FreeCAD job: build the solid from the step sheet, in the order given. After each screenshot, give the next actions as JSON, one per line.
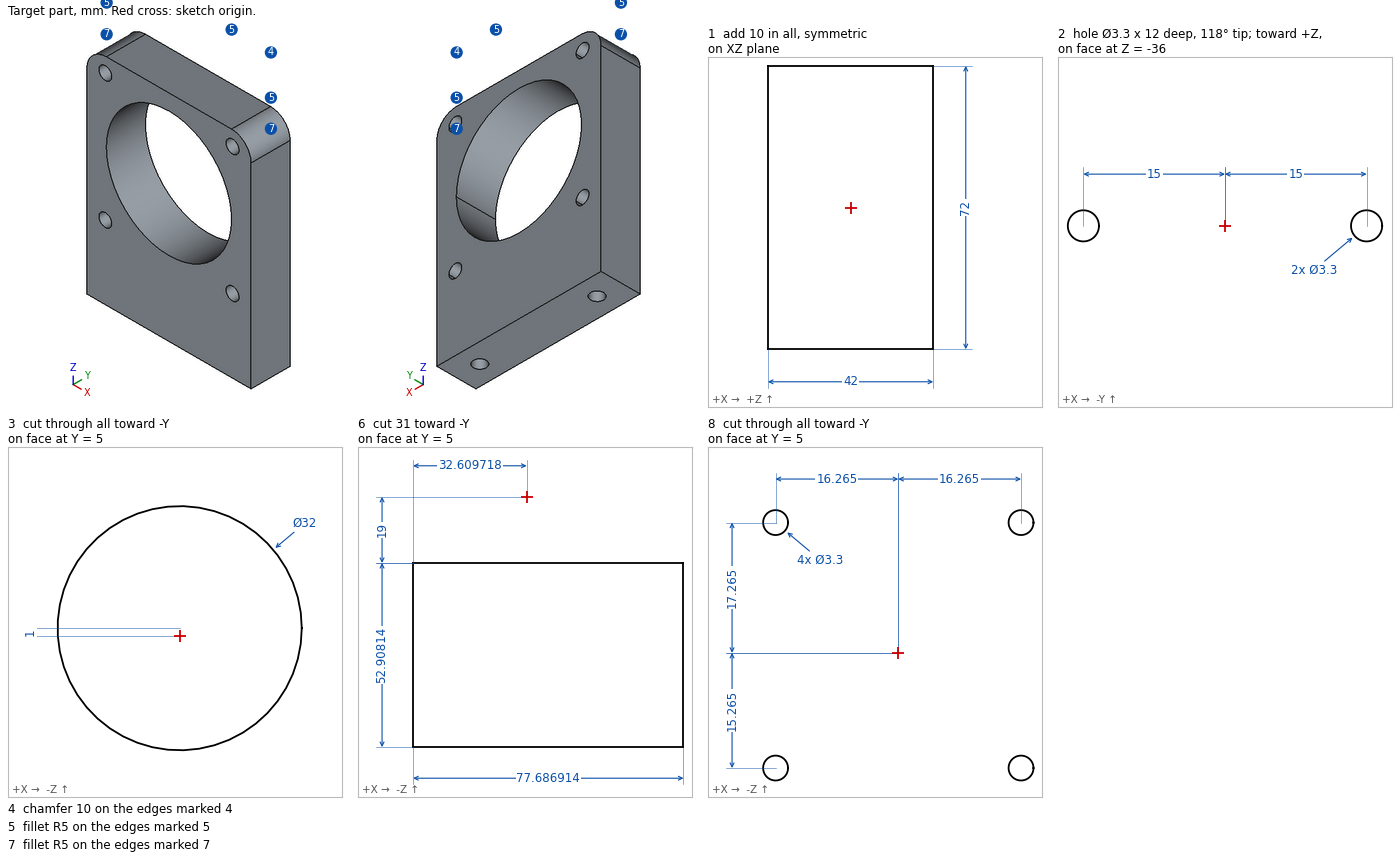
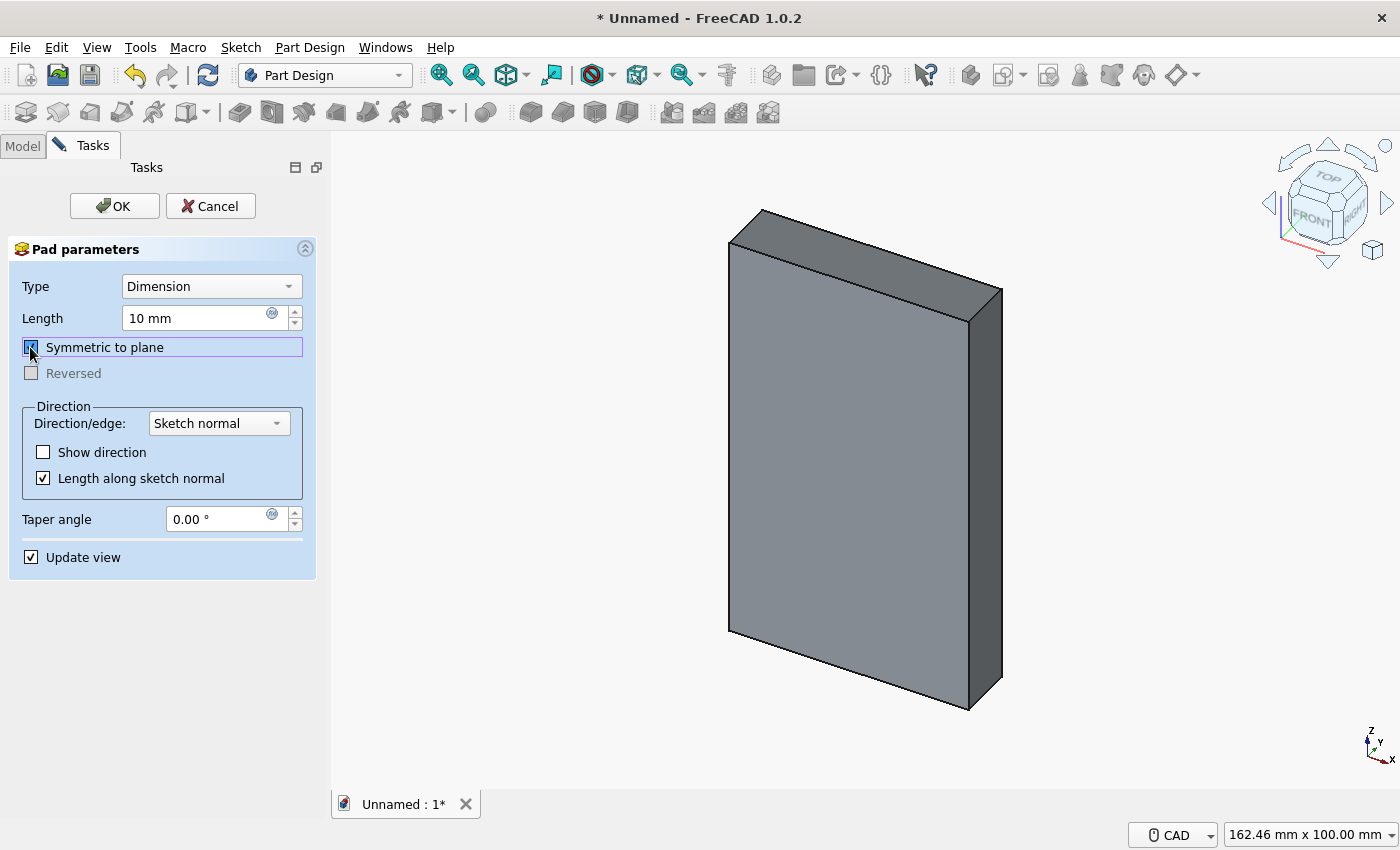
{"action": "left_click", "coordinate": [115, 206]}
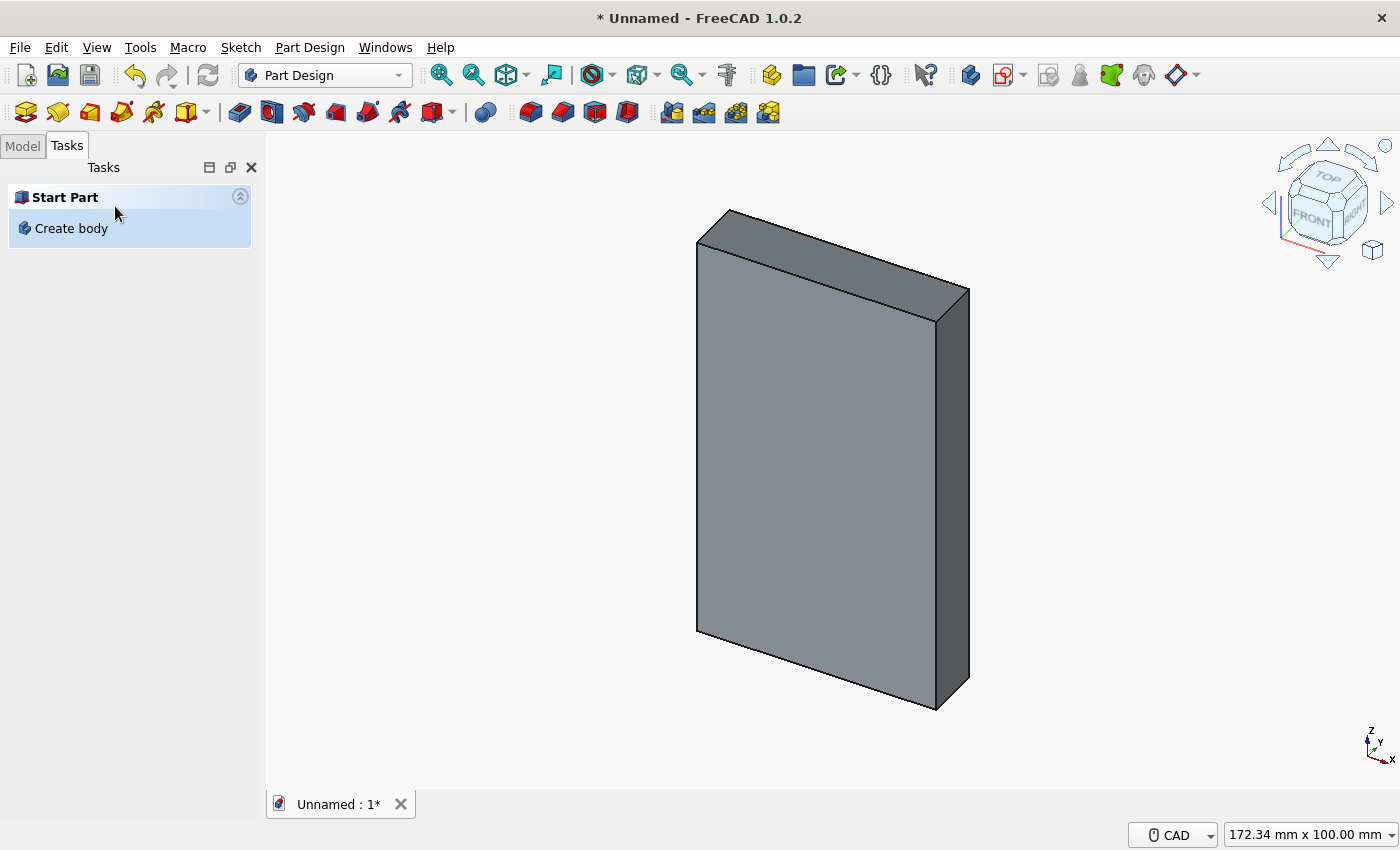
{"action": "key", "text": "5"}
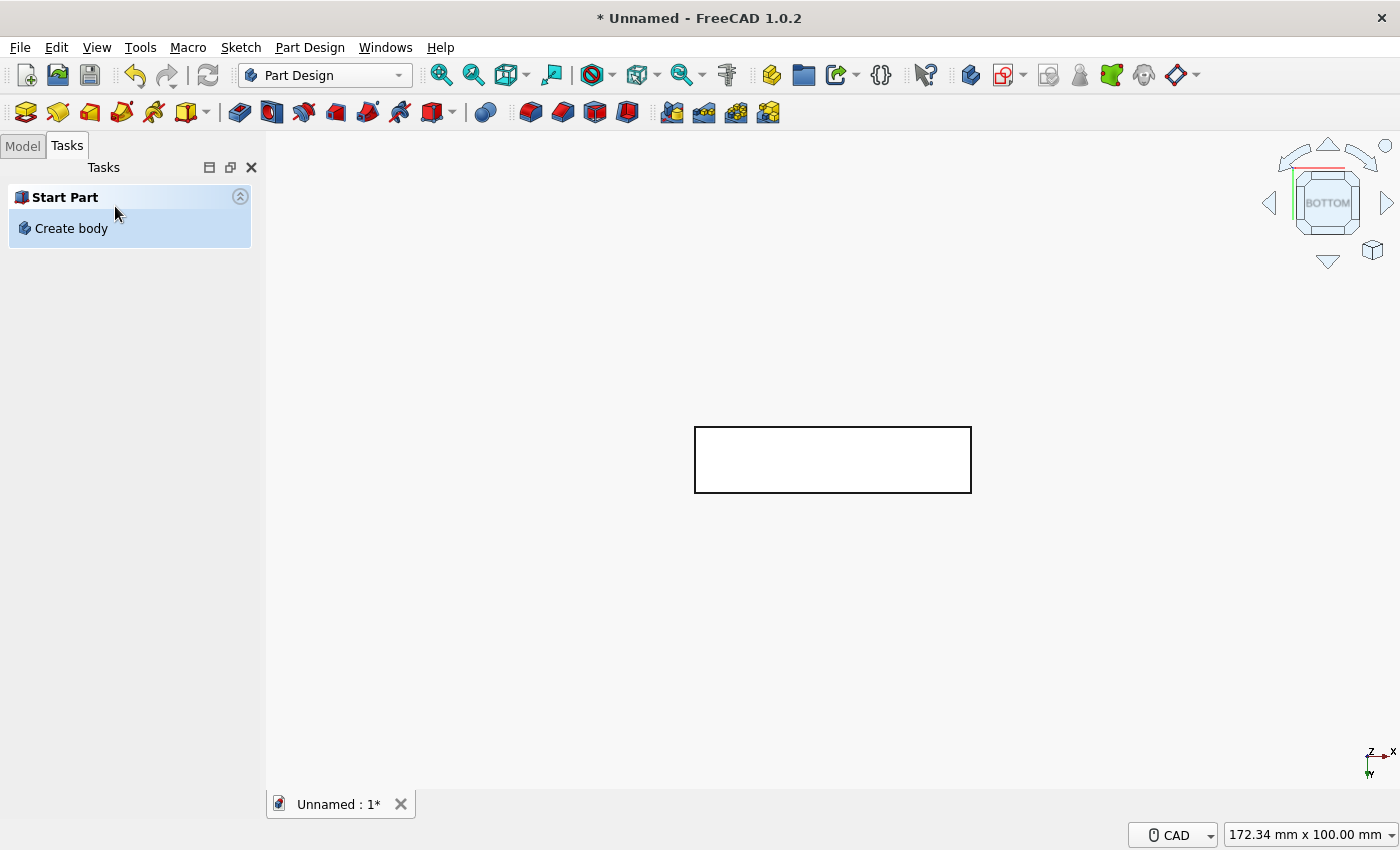
{"action": "left_click", "coordinate": [442, 76]}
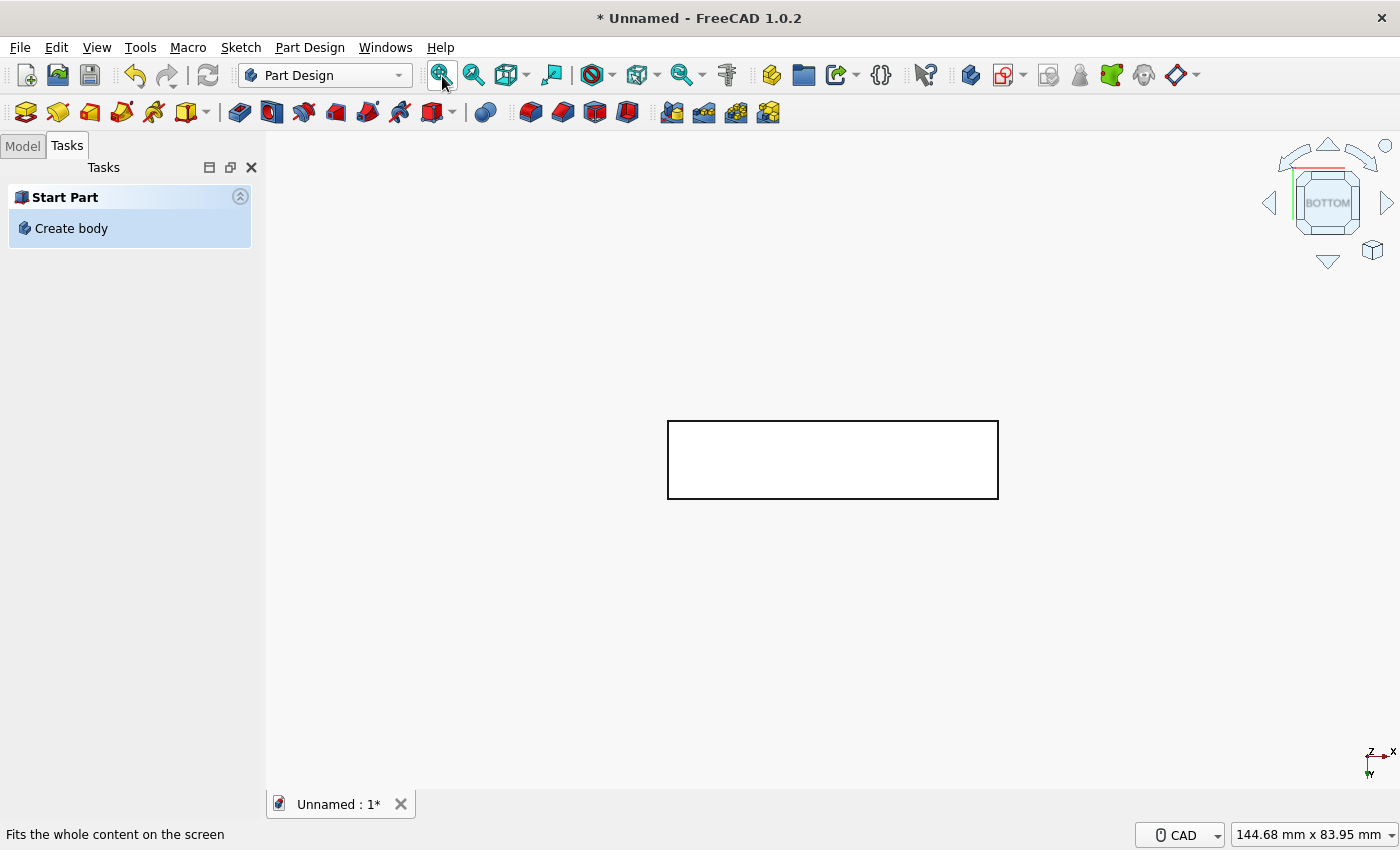
{"action": "left_click", "coordinate": [927, 459]}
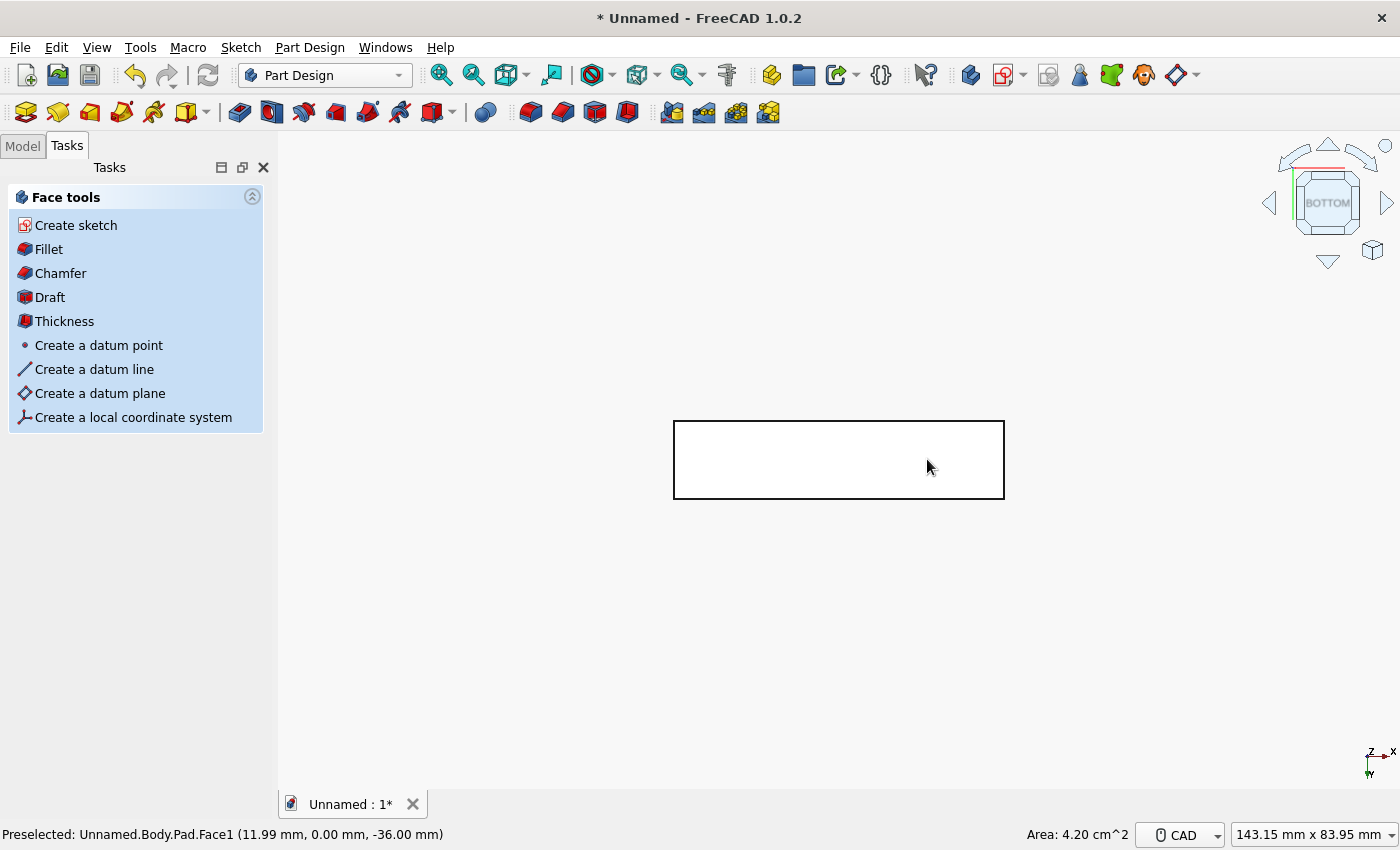
{"action": "left_click", "coordinate": [1004, 76]}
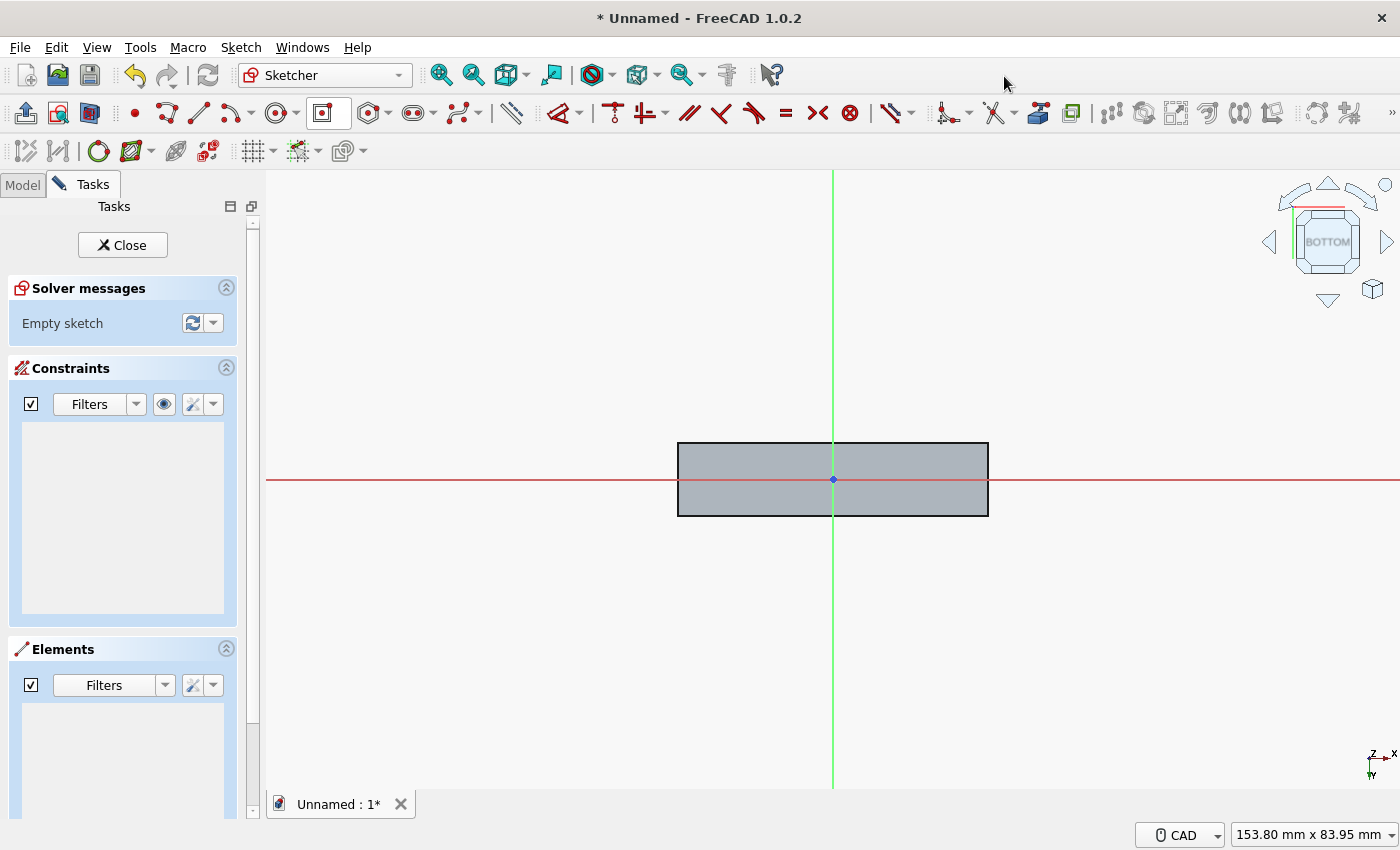
{"action": "scroll", "coordinate": [873, 479], "scroll_direction": "up", "scroll_amount": 5}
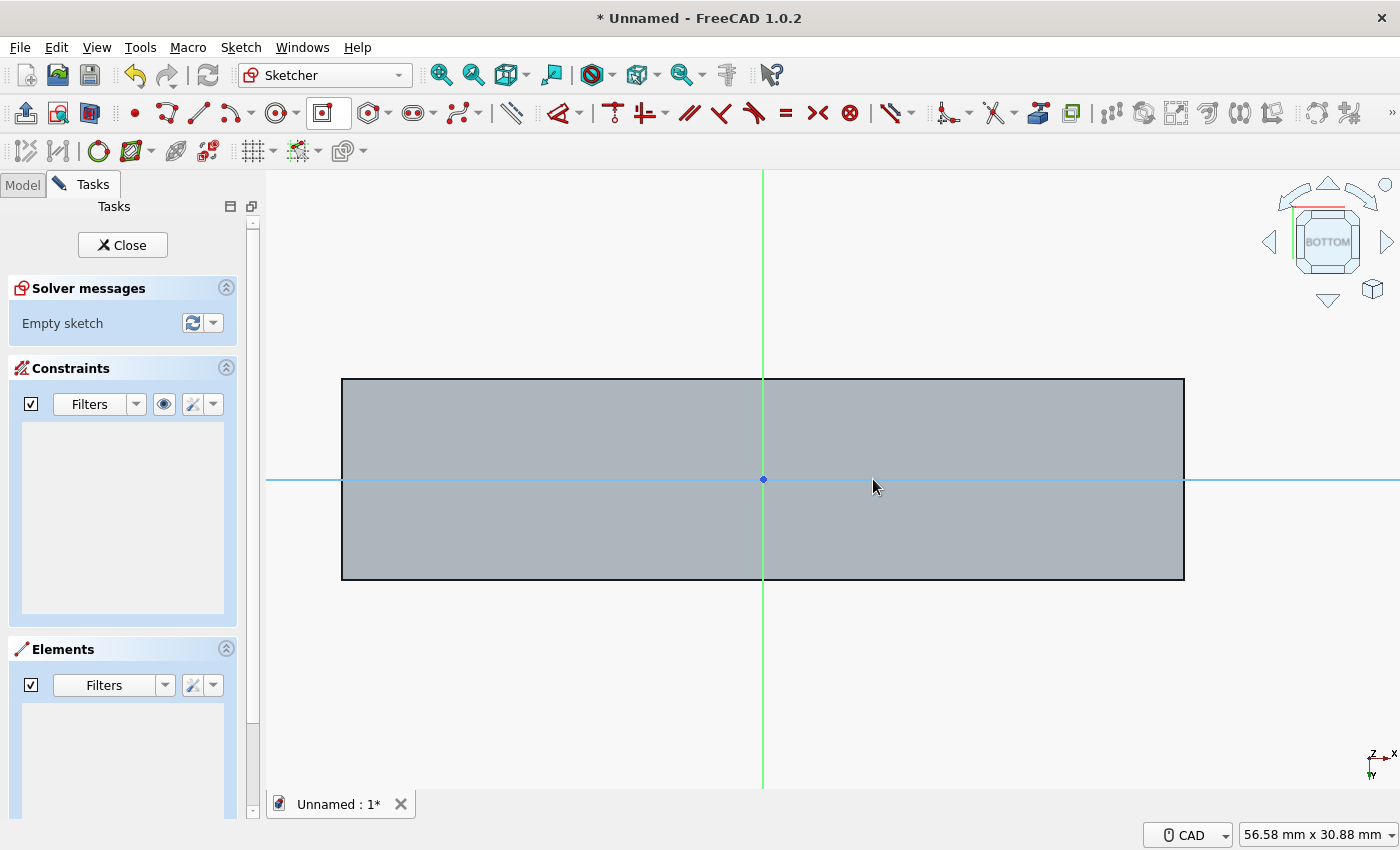
{"action": "left_click", "coordinate": [276, 114]}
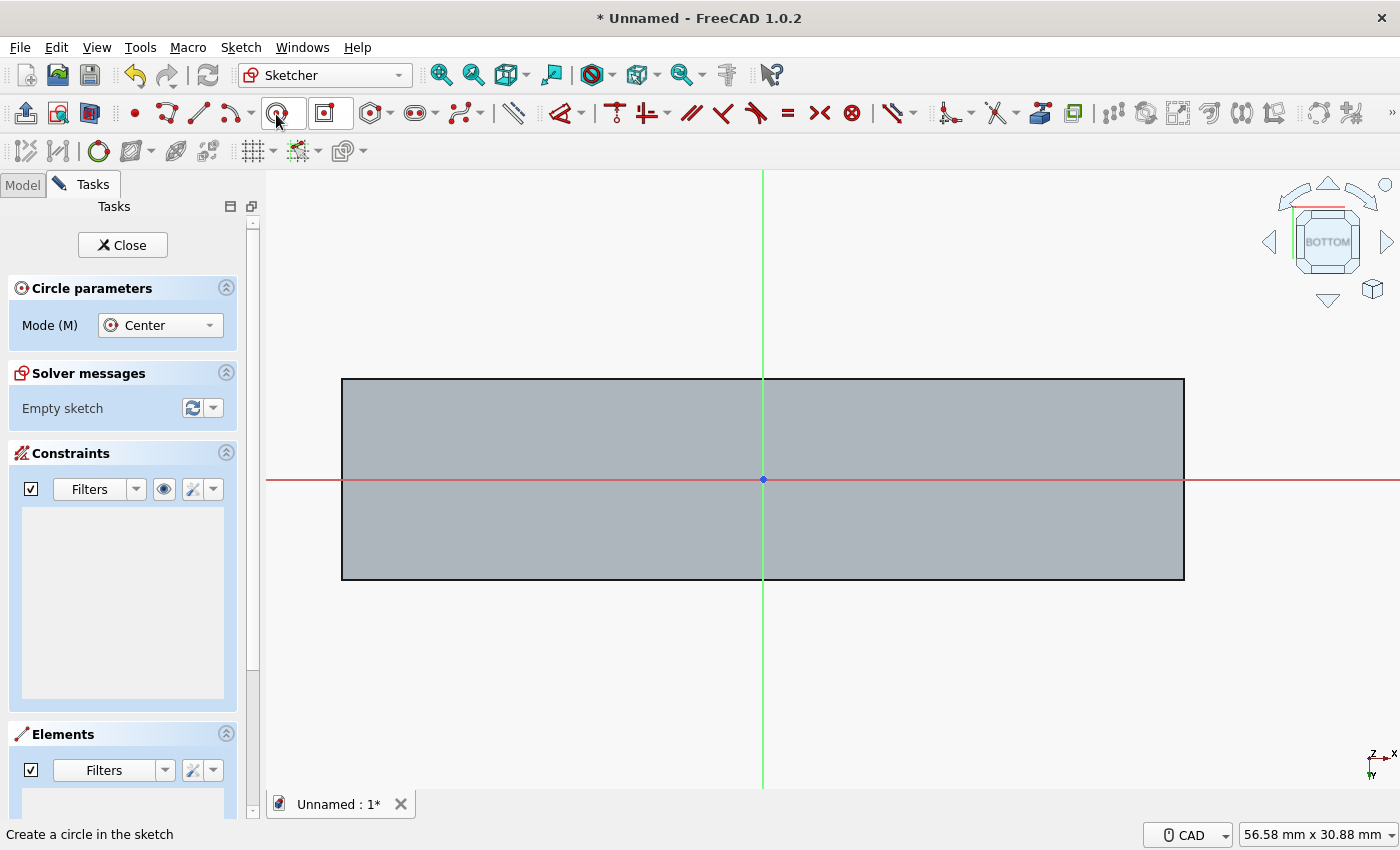
{"action": "left_click", "coordinate": [1064, 479]}
{"action": "left_click", "coordinate": [1087, 456]}